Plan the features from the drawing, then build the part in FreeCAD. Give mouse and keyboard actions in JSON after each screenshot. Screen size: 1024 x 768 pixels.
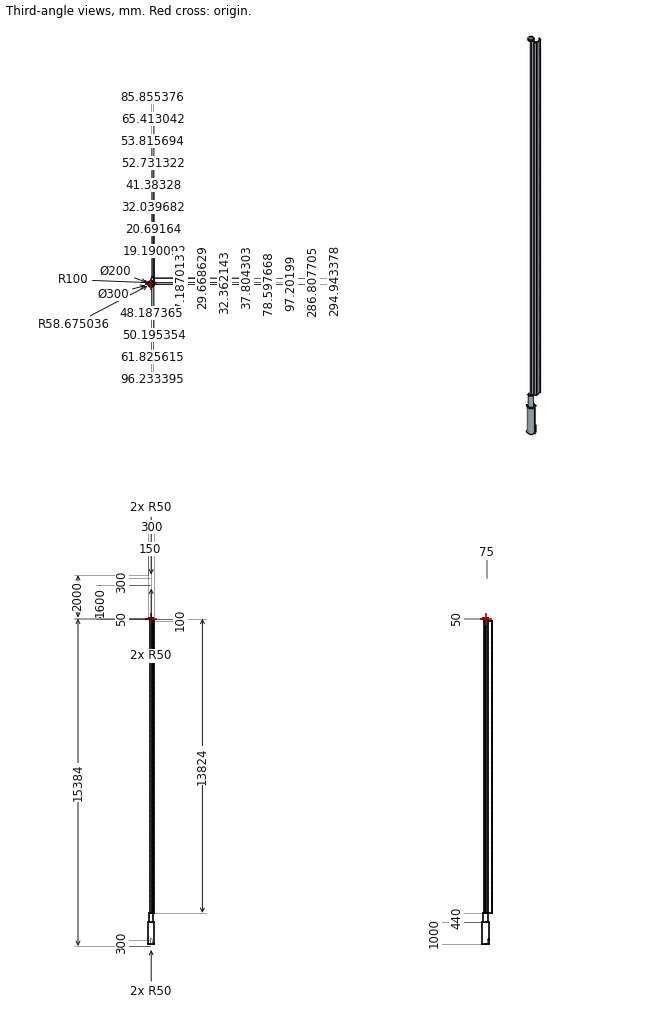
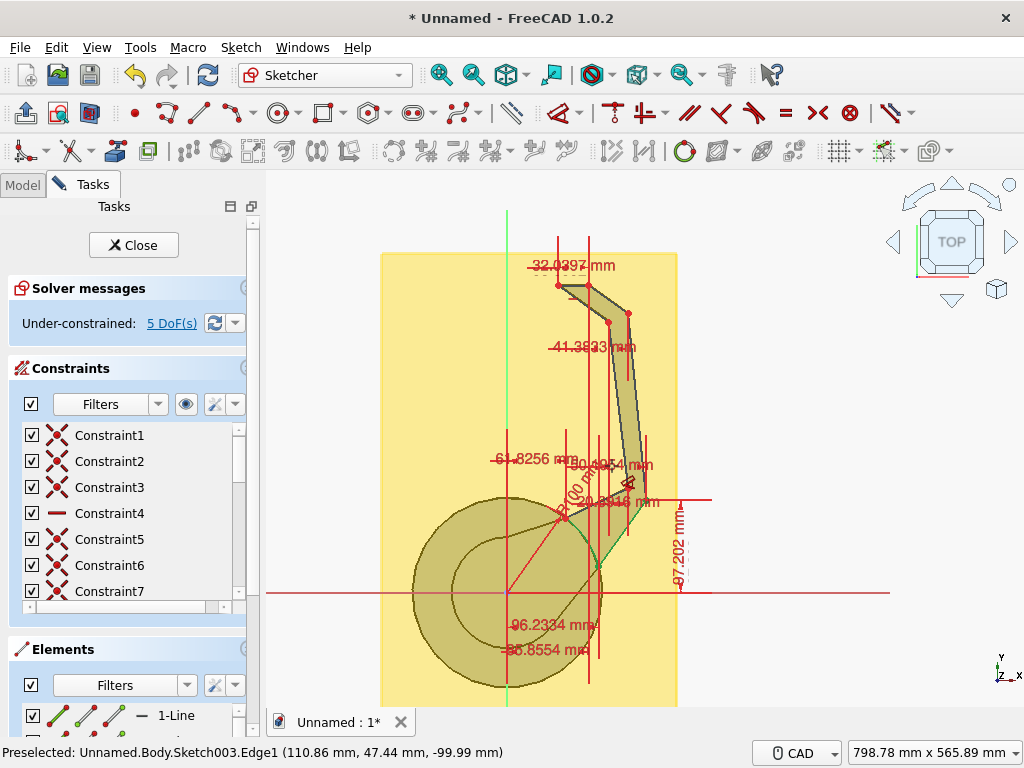
{"action": "scroll", "coordinate": [616, 305], "scroll_direction": "up", "scroll_amount": 2}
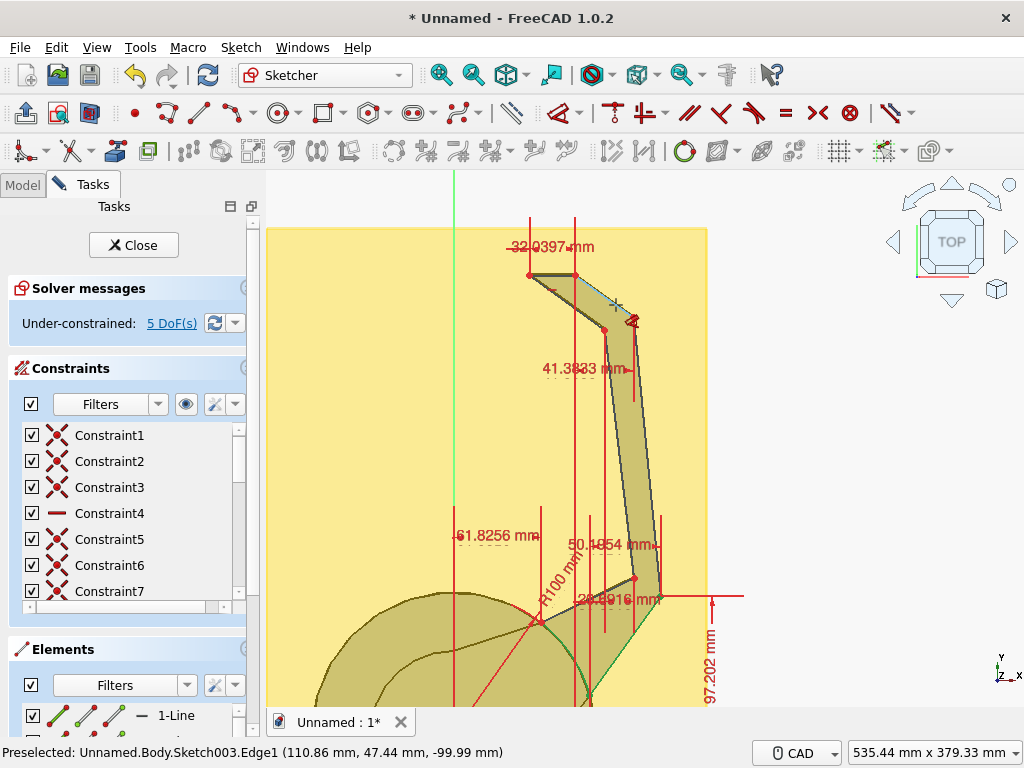
{"action": "left_click", "coordinate": [616, 305]}
{"action": "left_click", "coordinate": [668, 297]}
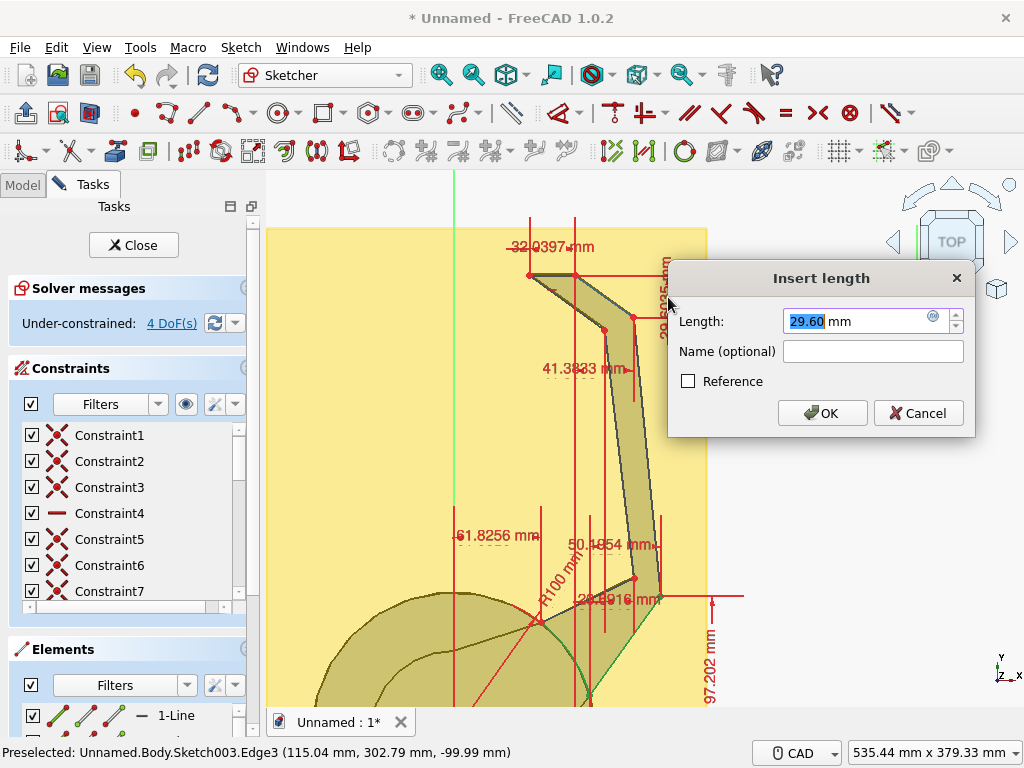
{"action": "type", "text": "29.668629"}
{"action": "key", "text": "Return"}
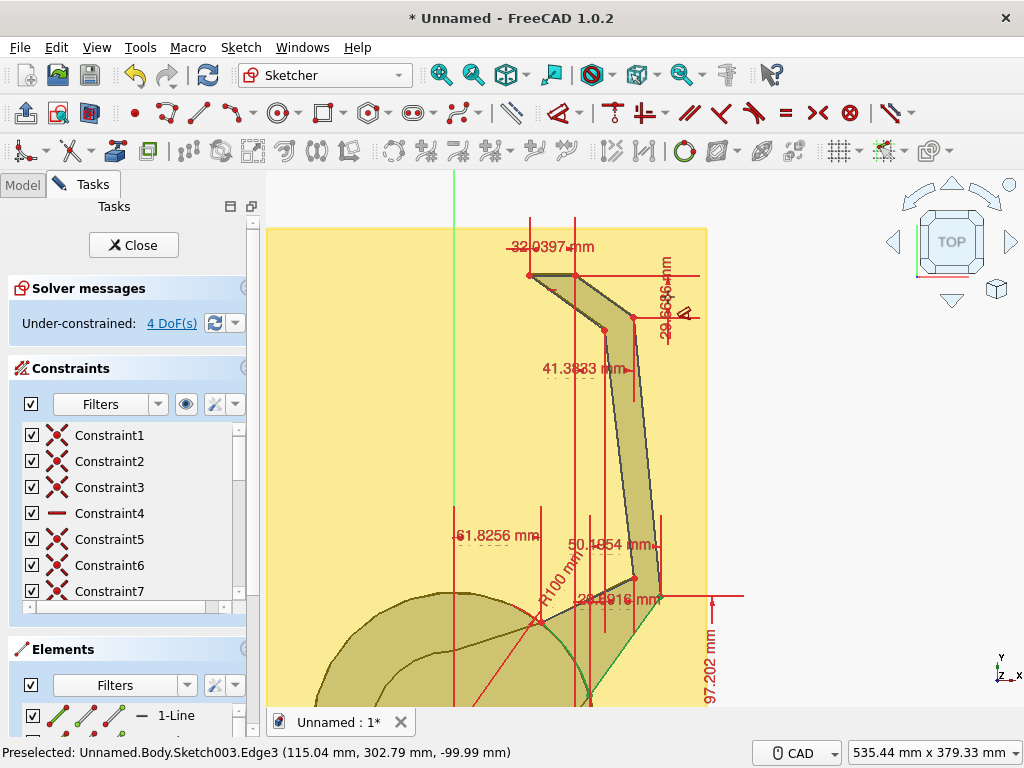
{"action": "left_click", "coordinate": [552, 292]}
{"action": "left_click", "coordinate": [567, 218]}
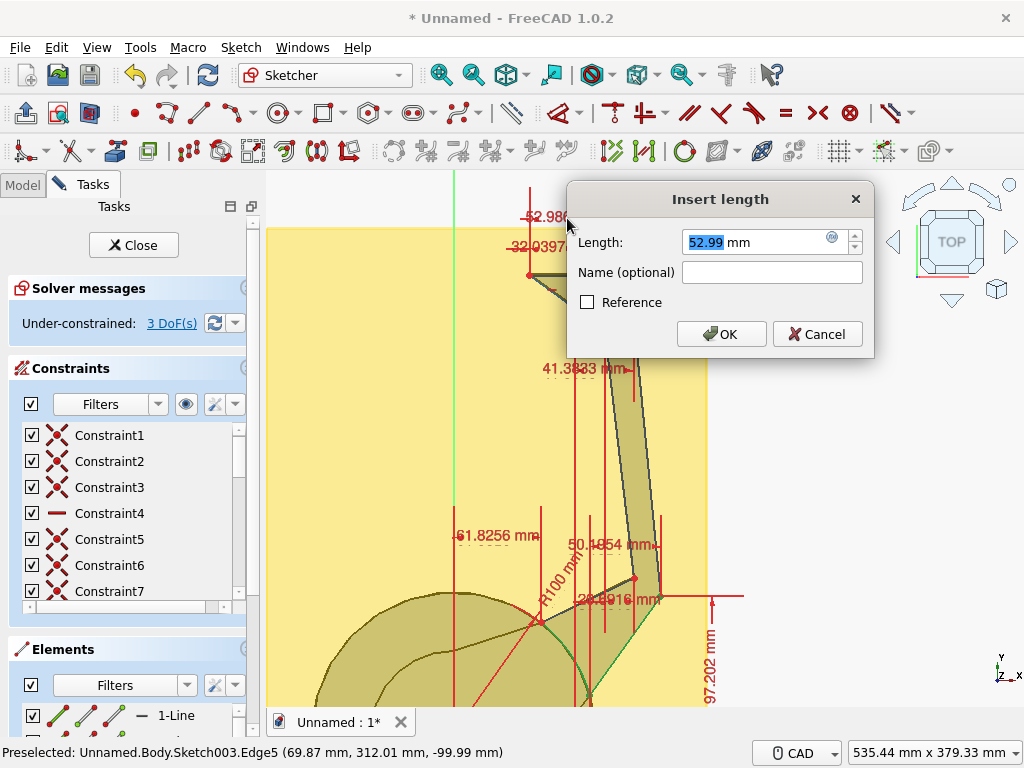
{"action": "type", "text": "52.731322"}
{"action": "key", "text": "Return"}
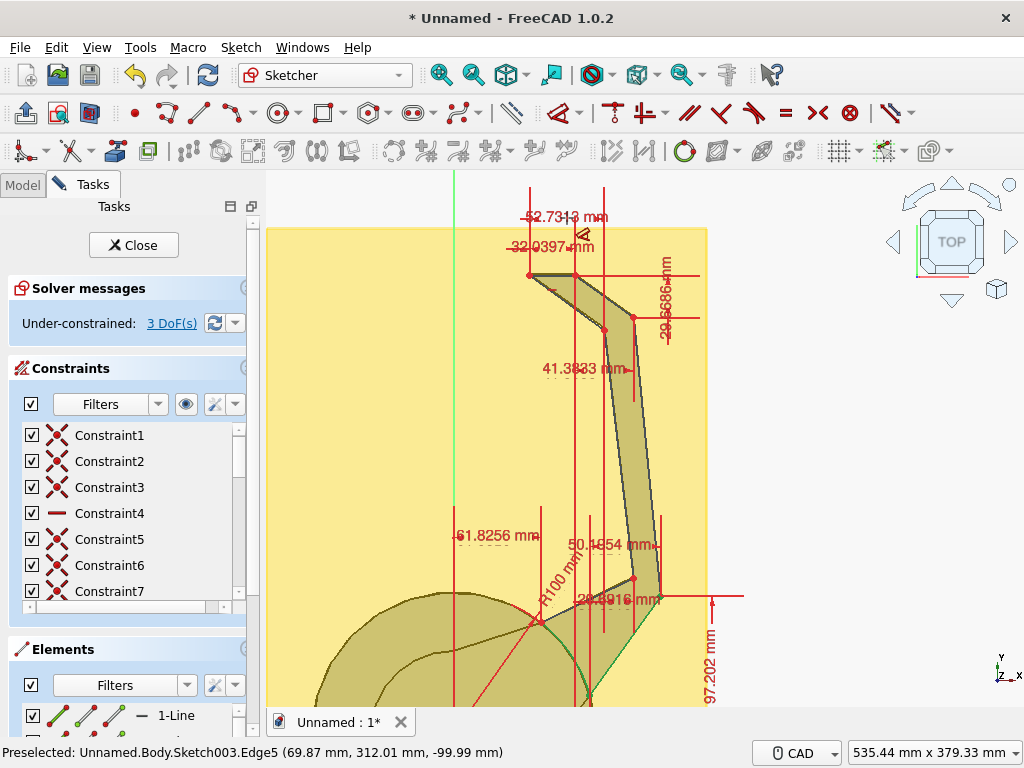
{"action": "left_click", "coordinate": [552, 292]}
{"action": "left_click", "coordinate": [496, 303]}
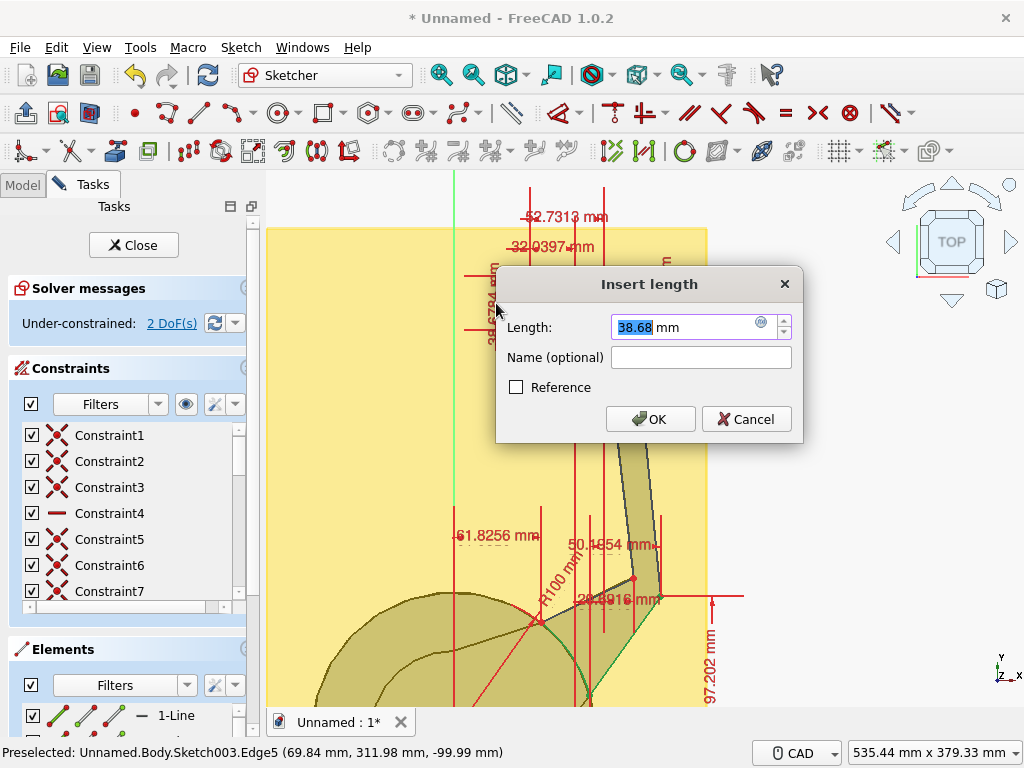
{"action": "type", "text": "37.804303"}
{"action": "key", "text": "Return"}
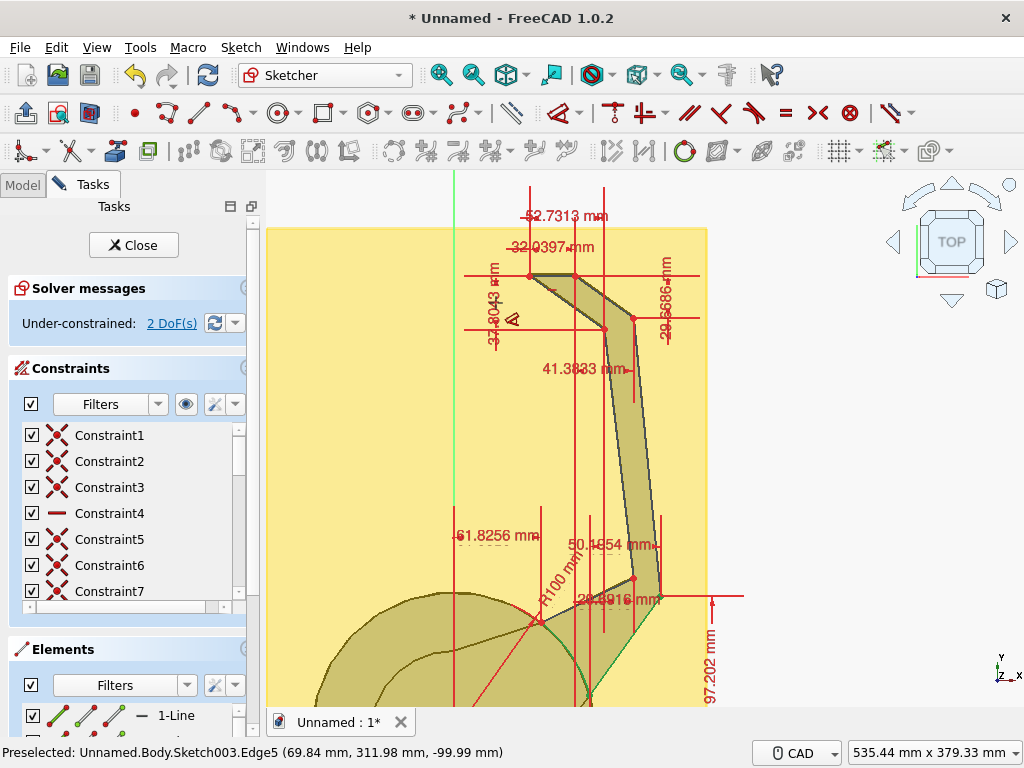
{"action": "left_click", "coordinate": [606, 592]}
{"action": "left_click", "coordinate": [507, 601]}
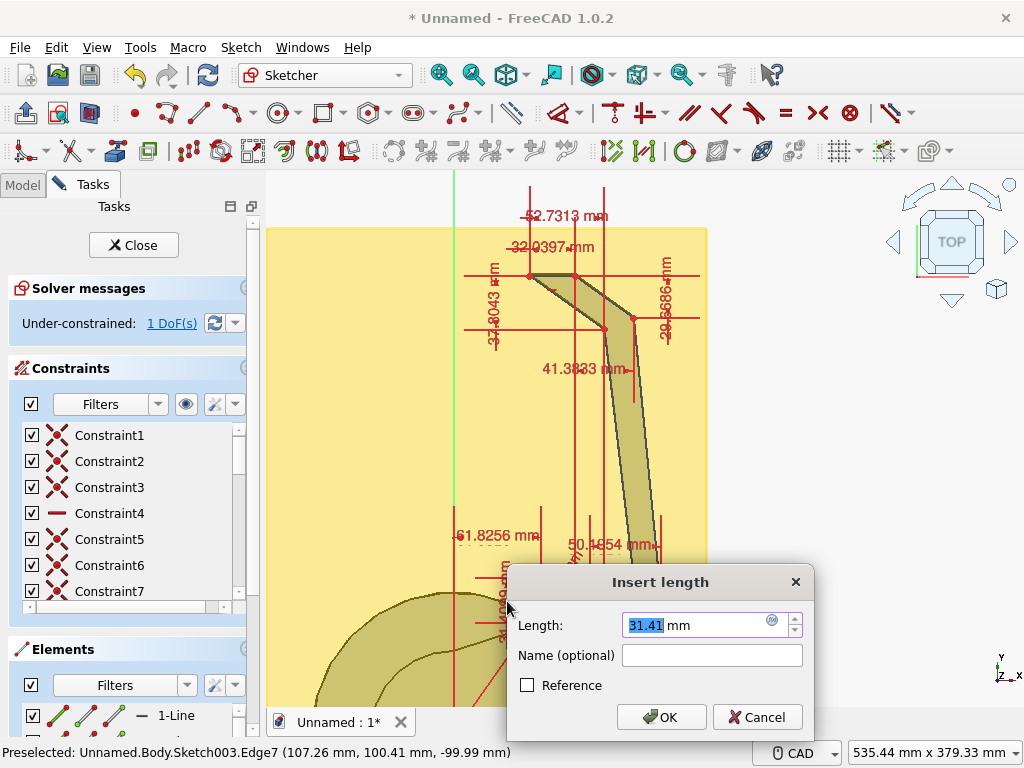
{"action": "type", "text": "32.362143"}
{"action": "key", "text": "Return"}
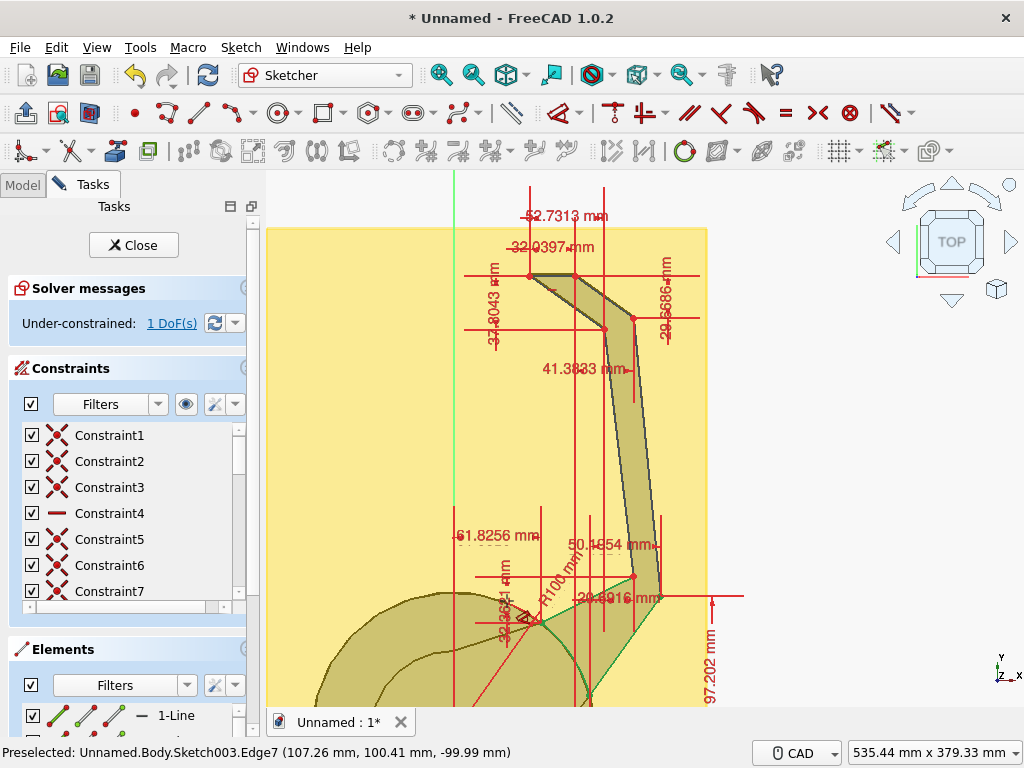
{"action": "left_click", "coordinate": [634, 318]}
{"action": "left_click", "coordinate": [420, 499]}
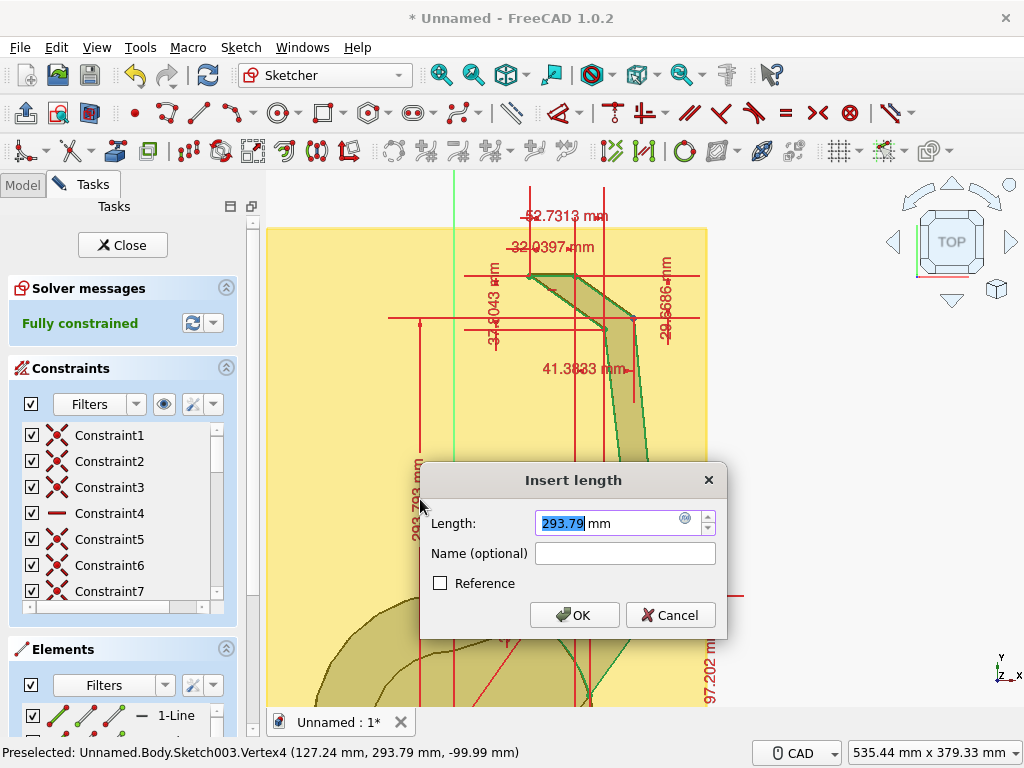
{"action": "type", "text": "294.943378"}
{"action": "key", "text": "Return"}
{"action": "key", "text": "Escape"}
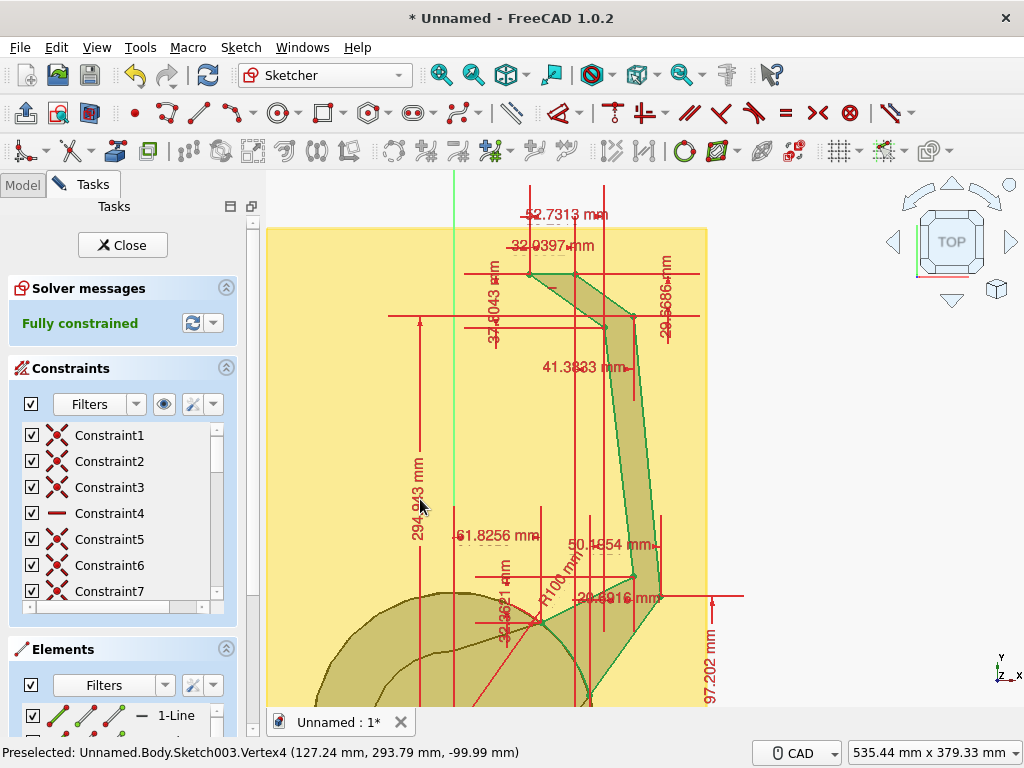
{"action": "left_click", "coordinate": [123, 245]}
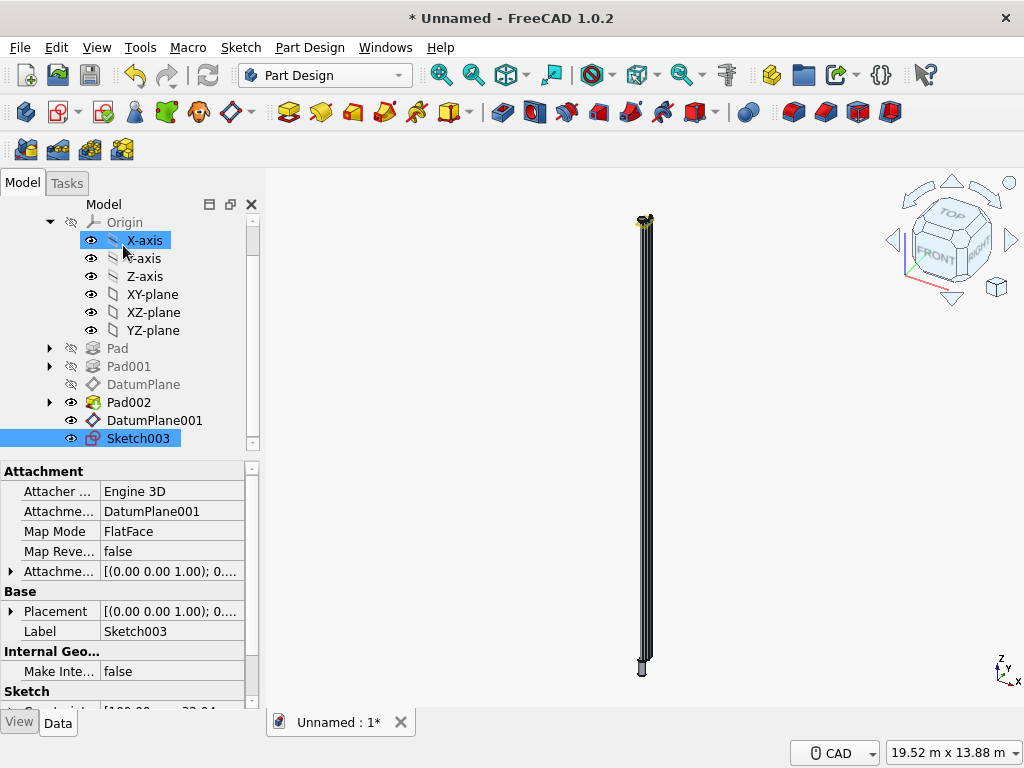
{"action": "left_click", "coordinate": [504, 112]}